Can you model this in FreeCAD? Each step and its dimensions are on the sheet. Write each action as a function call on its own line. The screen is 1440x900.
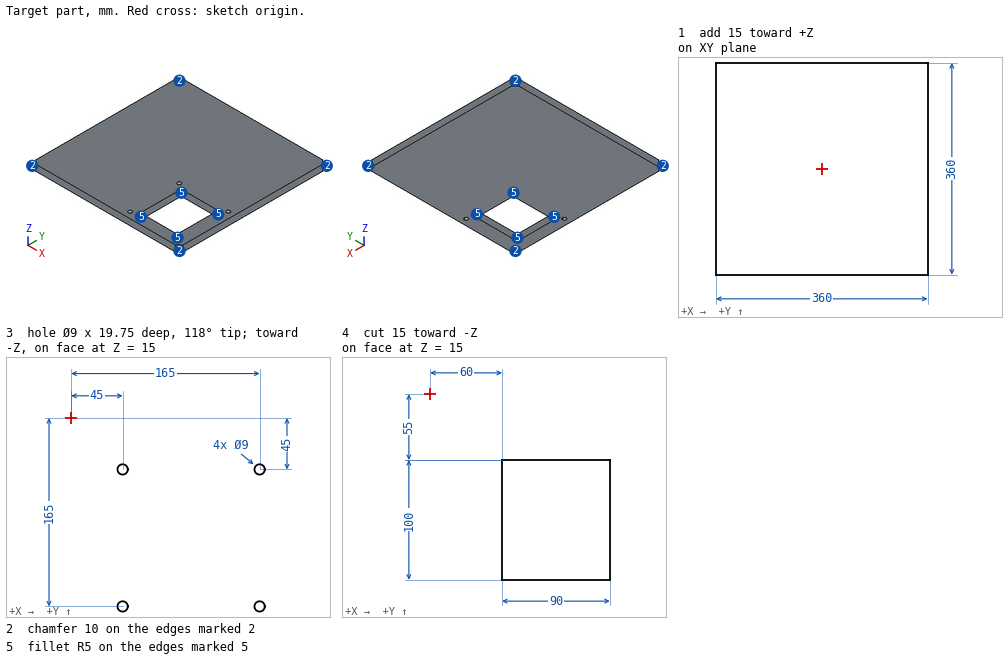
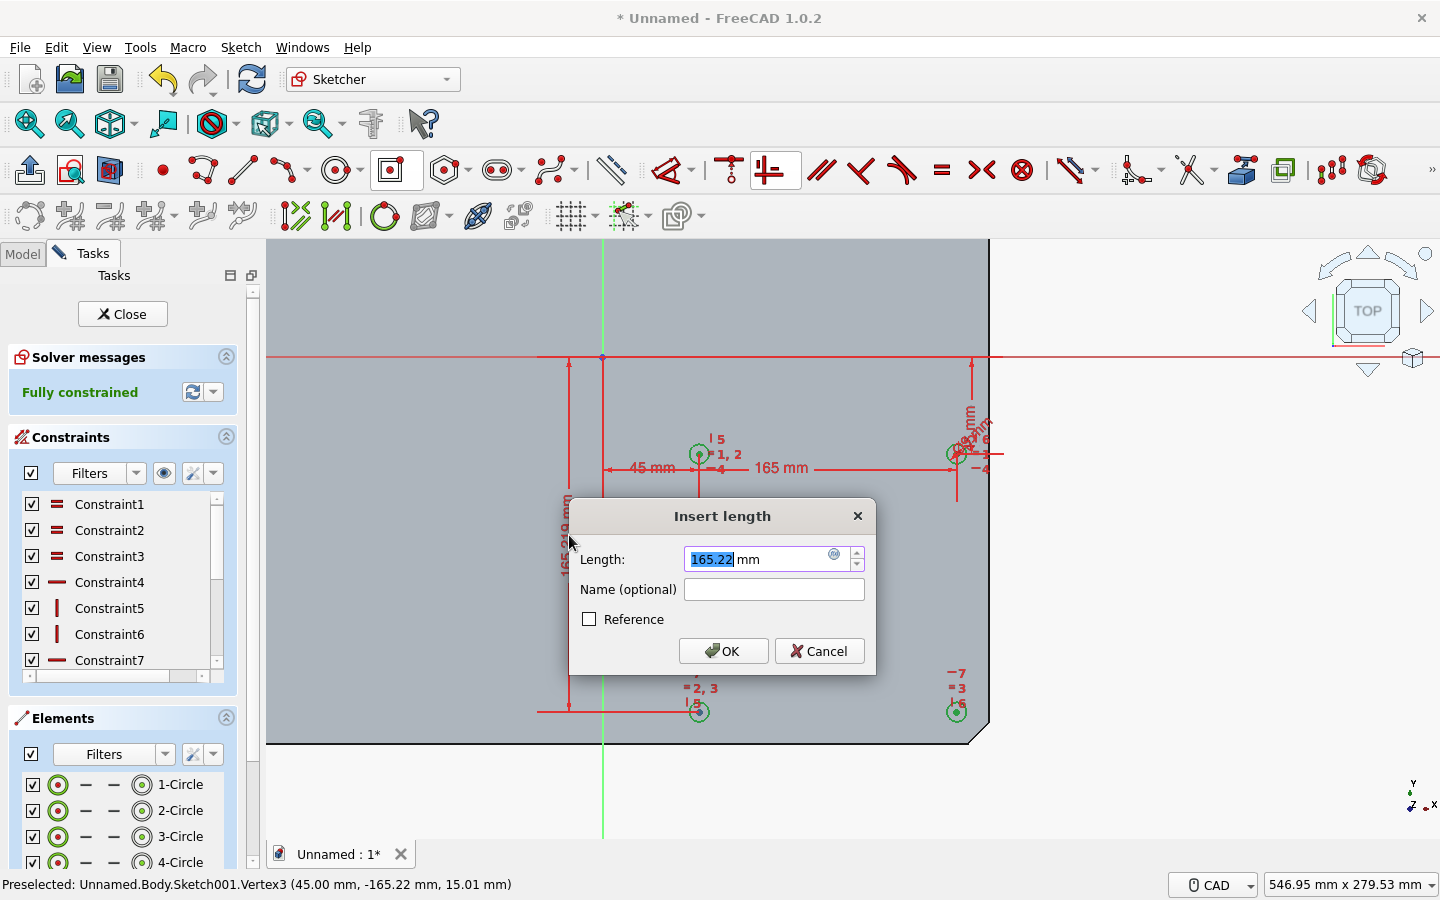
text(165)
key(Return)
key(Escape)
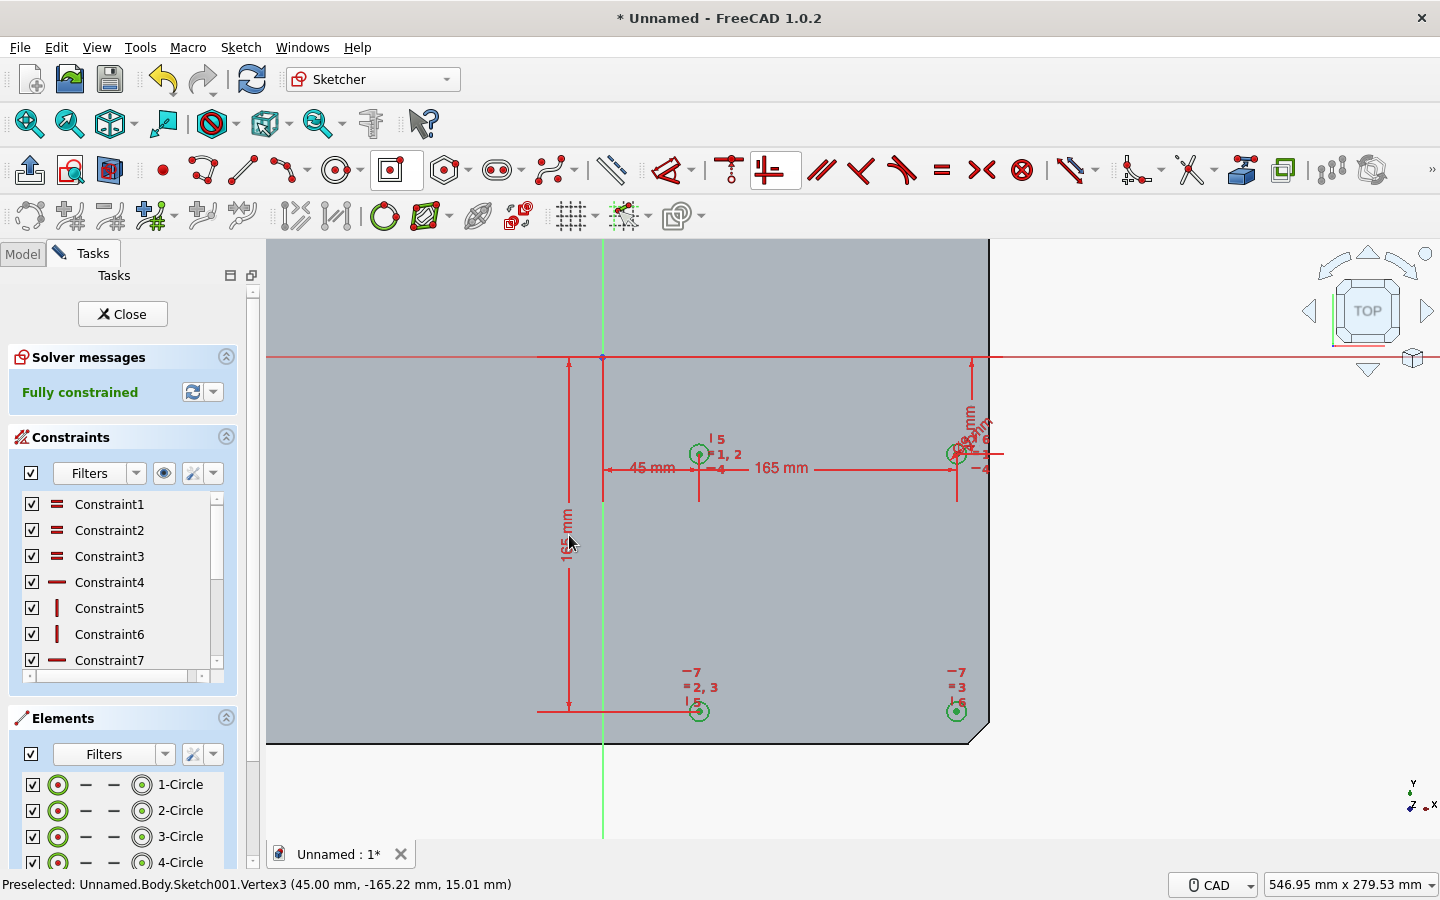
click(123, 314)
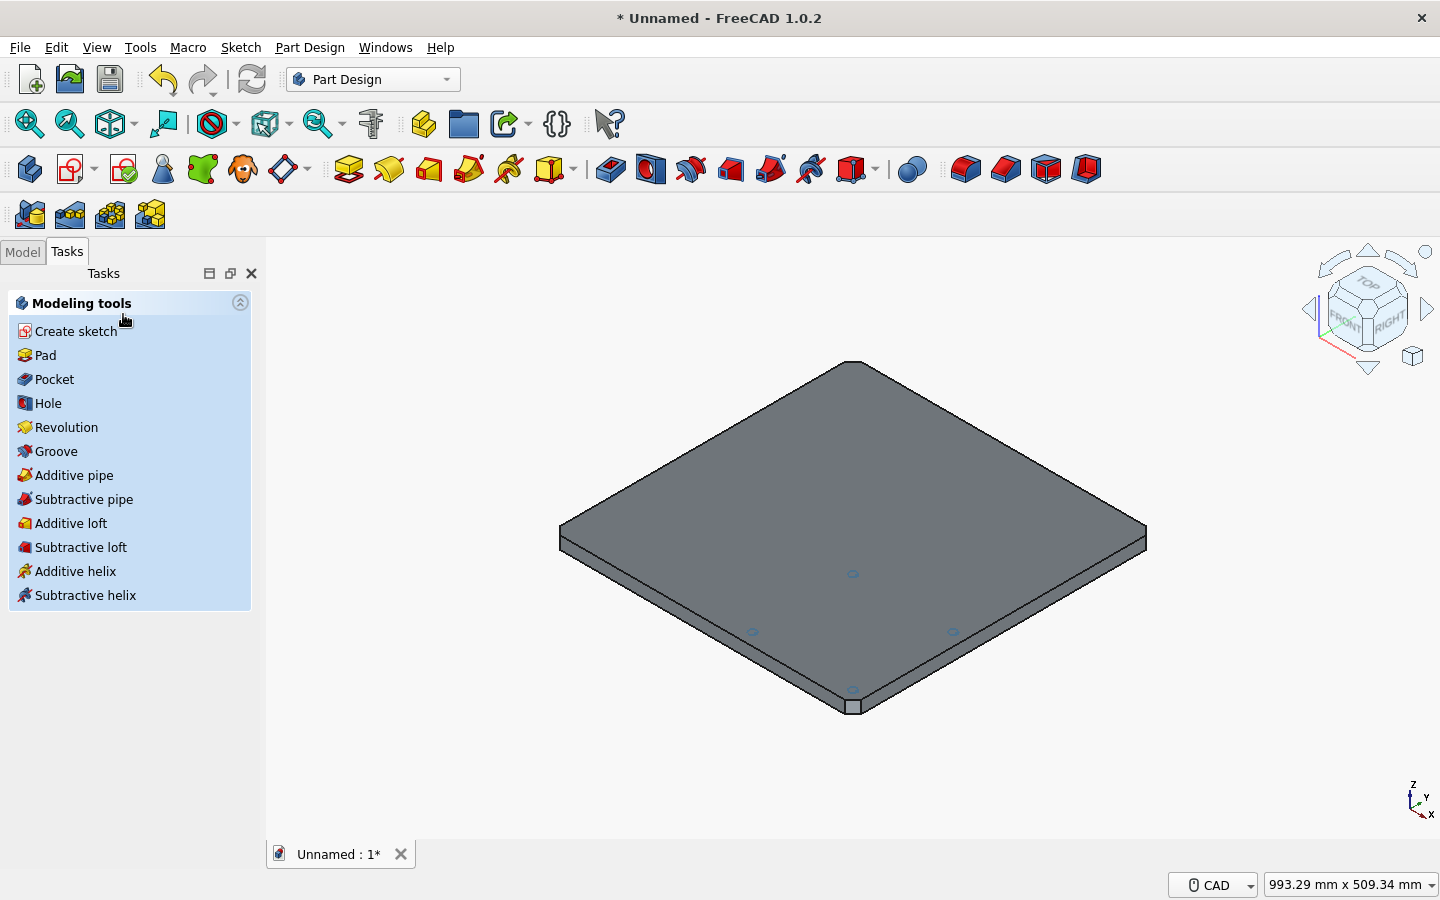
click(652, 170)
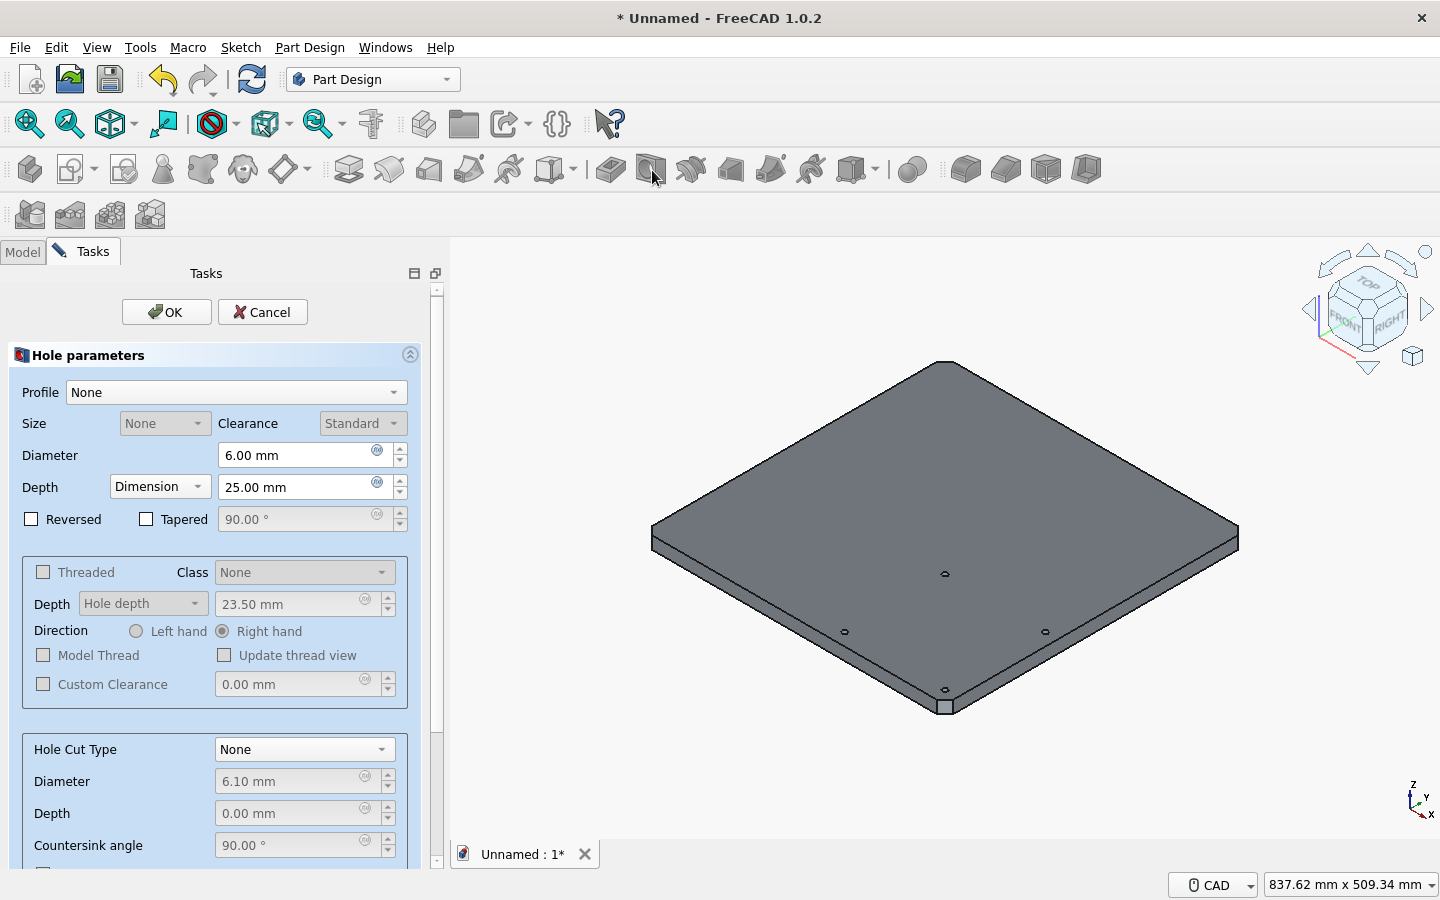
triple_click(305, 455)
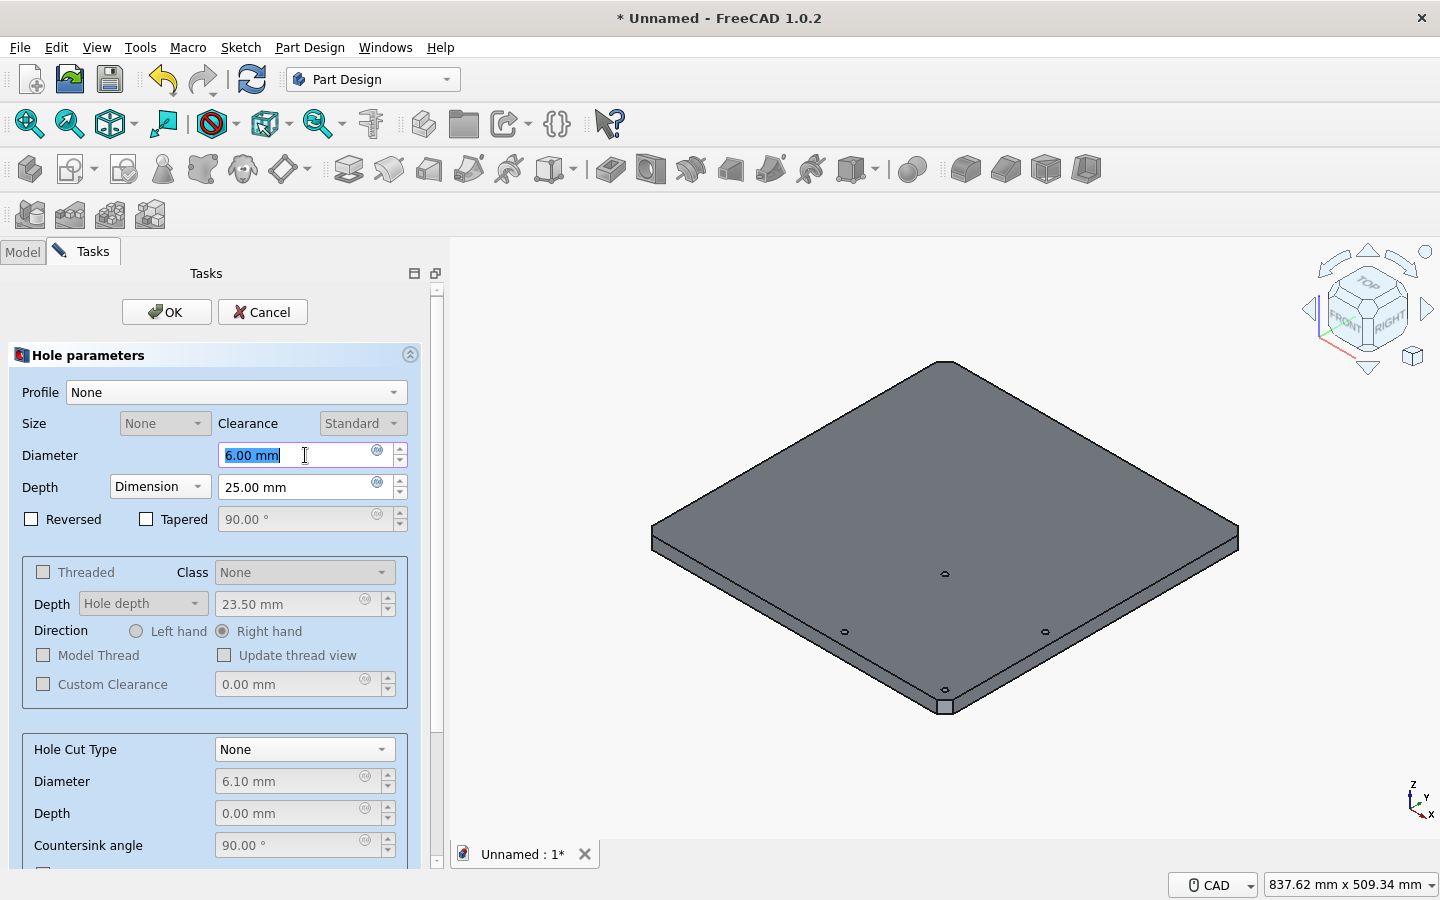
text(9)
key(Tab)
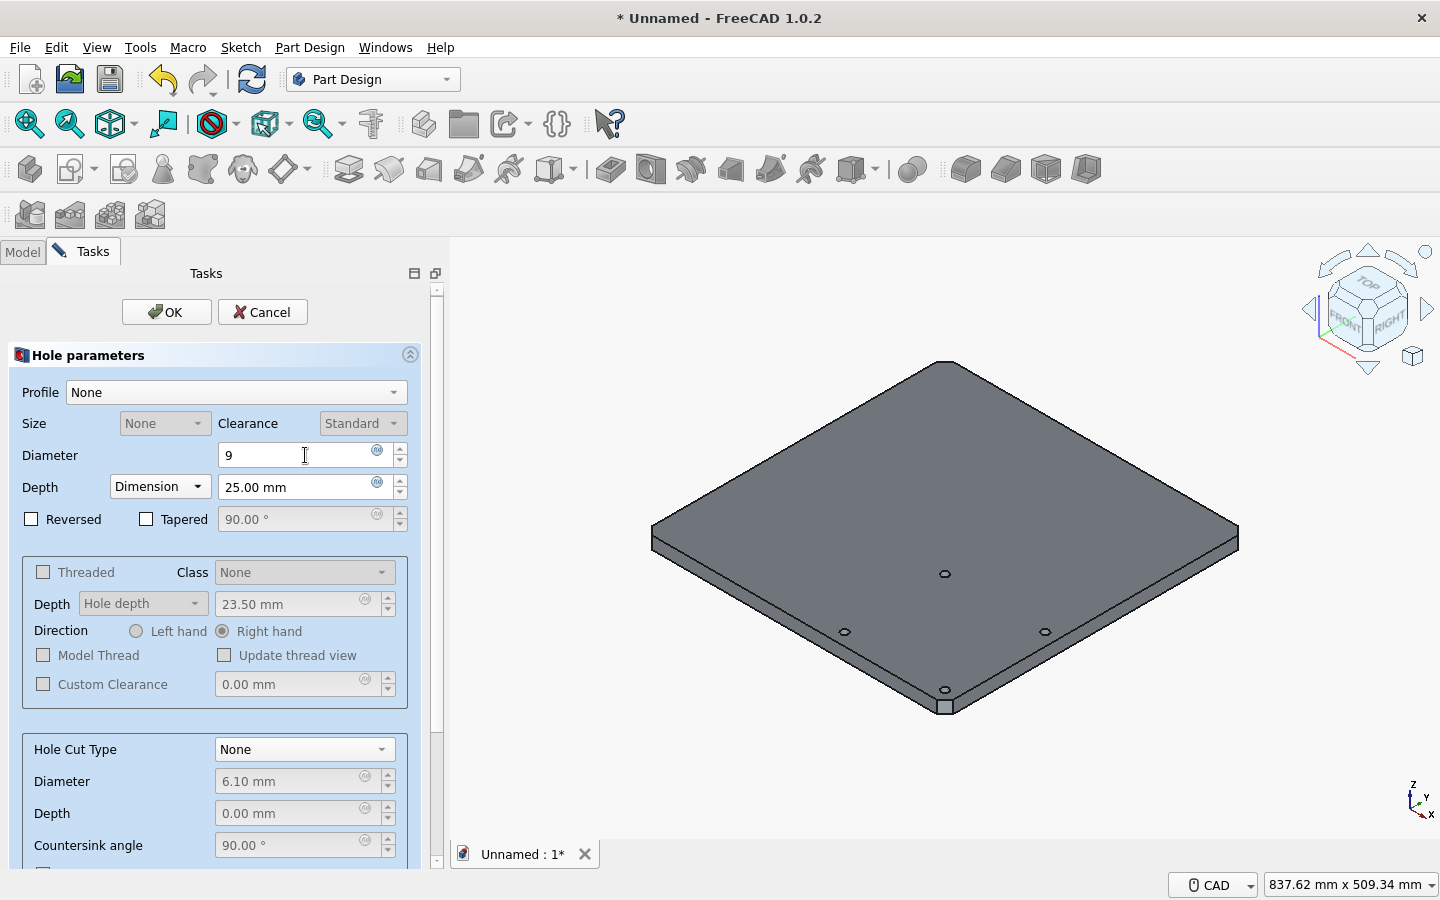
triple_click(305, 487)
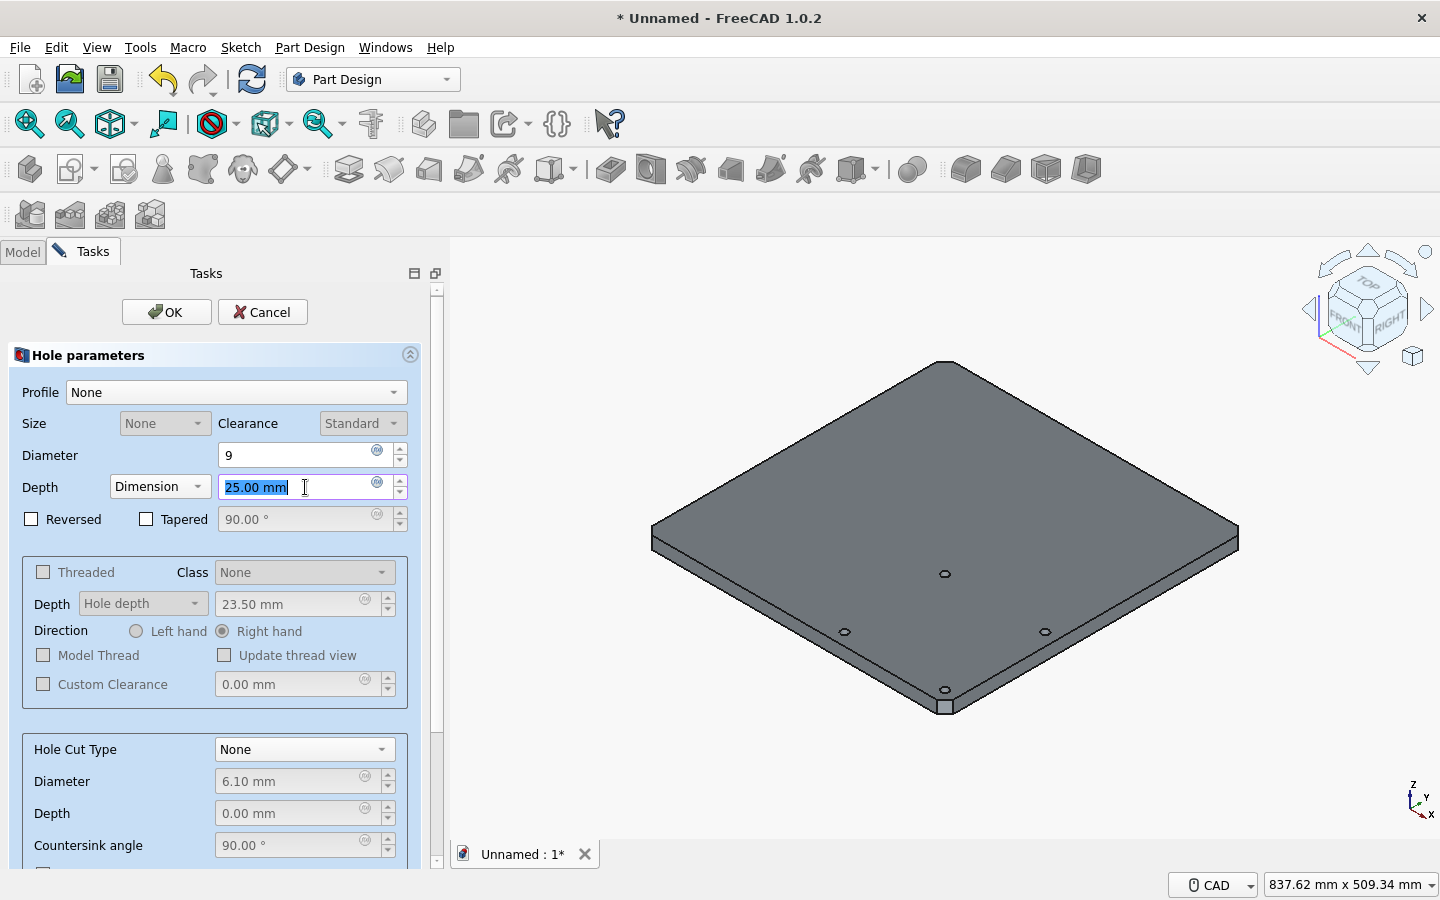
text(19.75)
key(Tab)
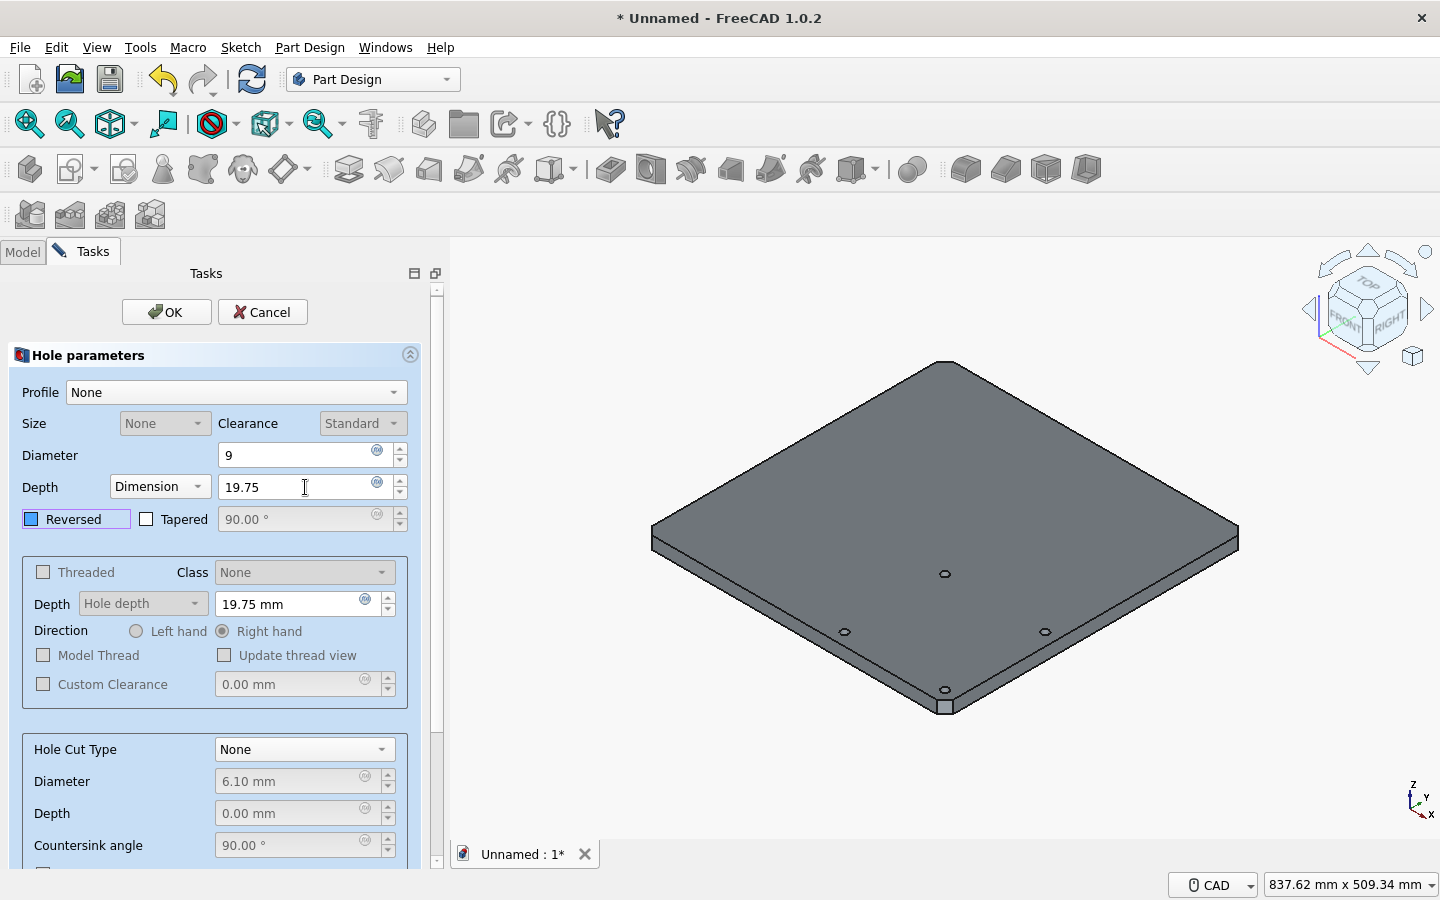
click(167, 312)